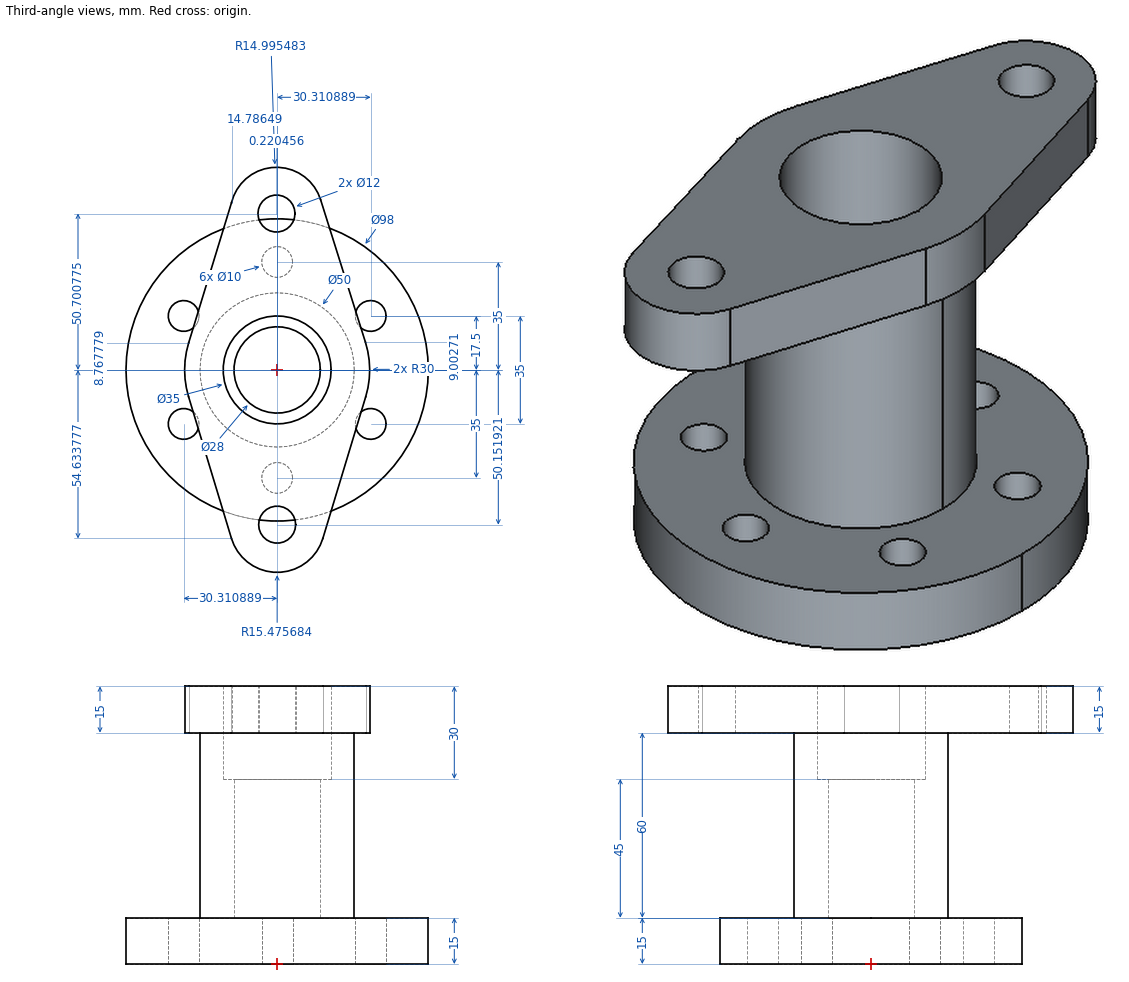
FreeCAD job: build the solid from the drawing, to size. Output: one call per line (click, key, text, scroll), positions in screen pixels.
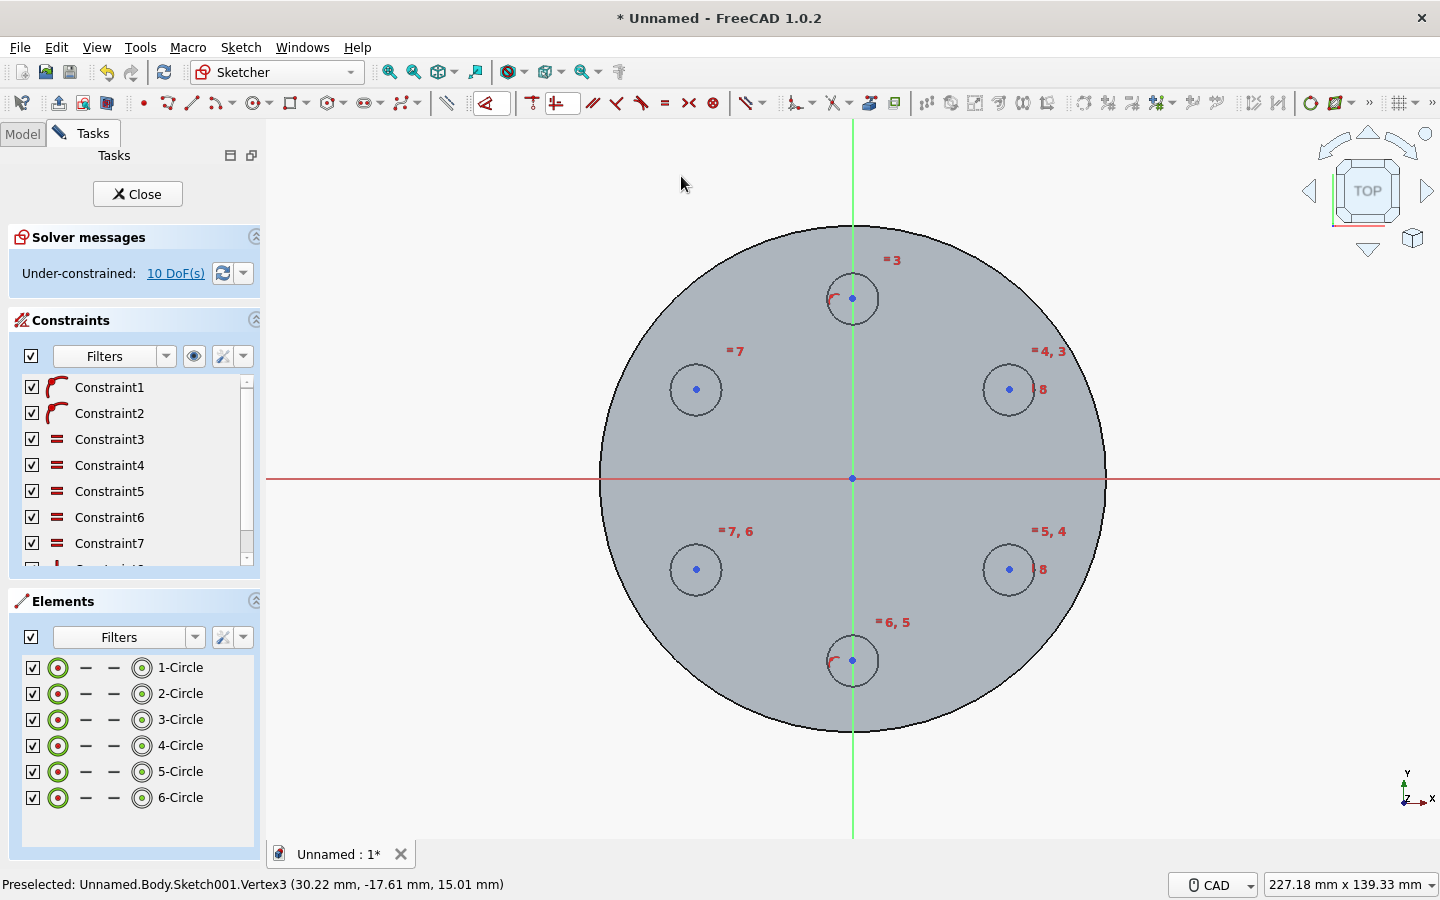
click(1009, 570)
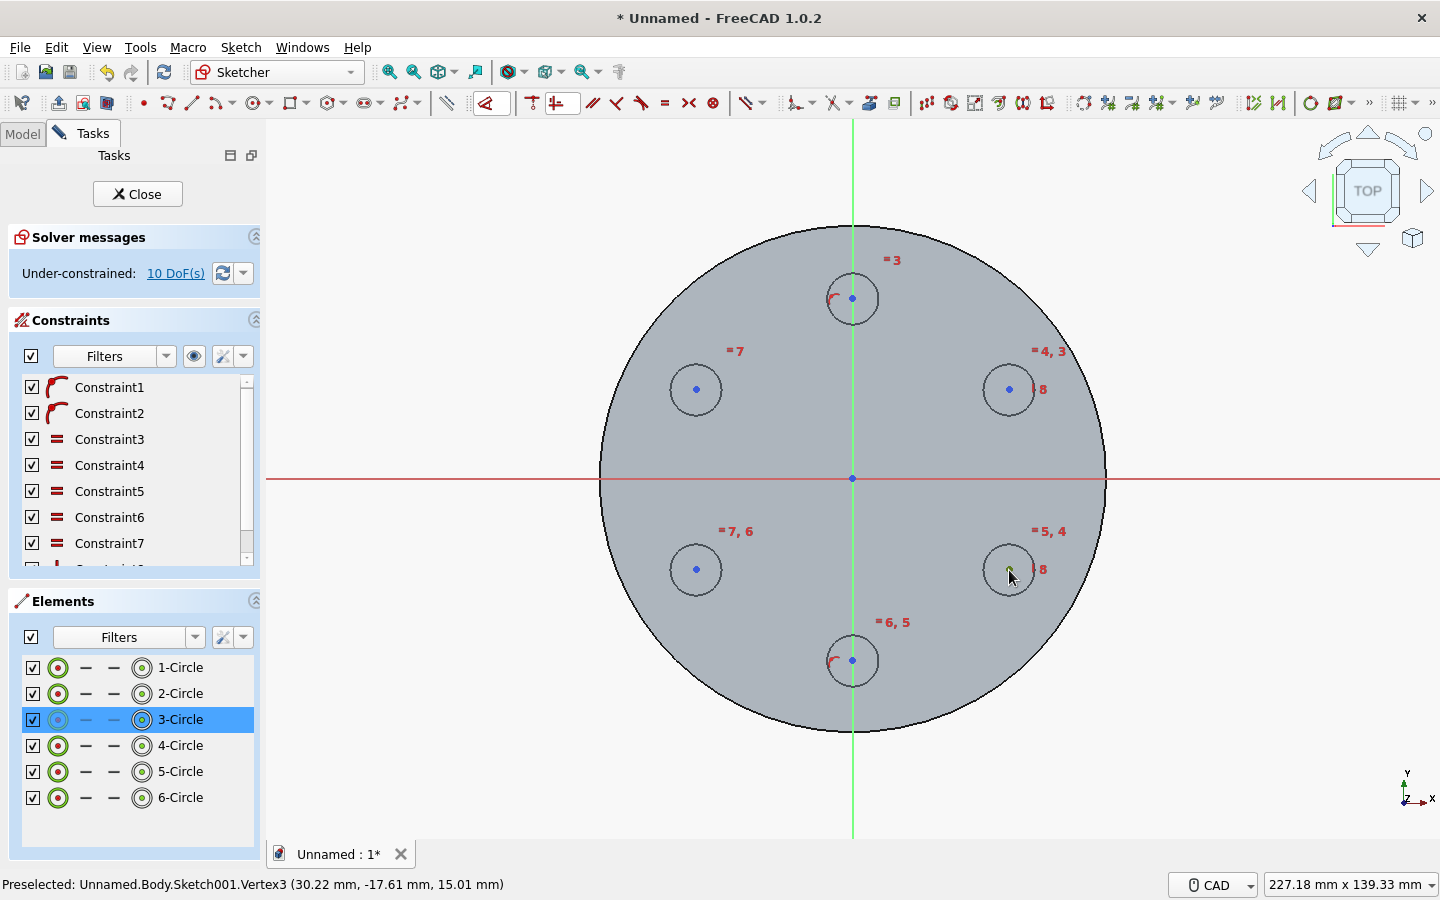
click(696, 570)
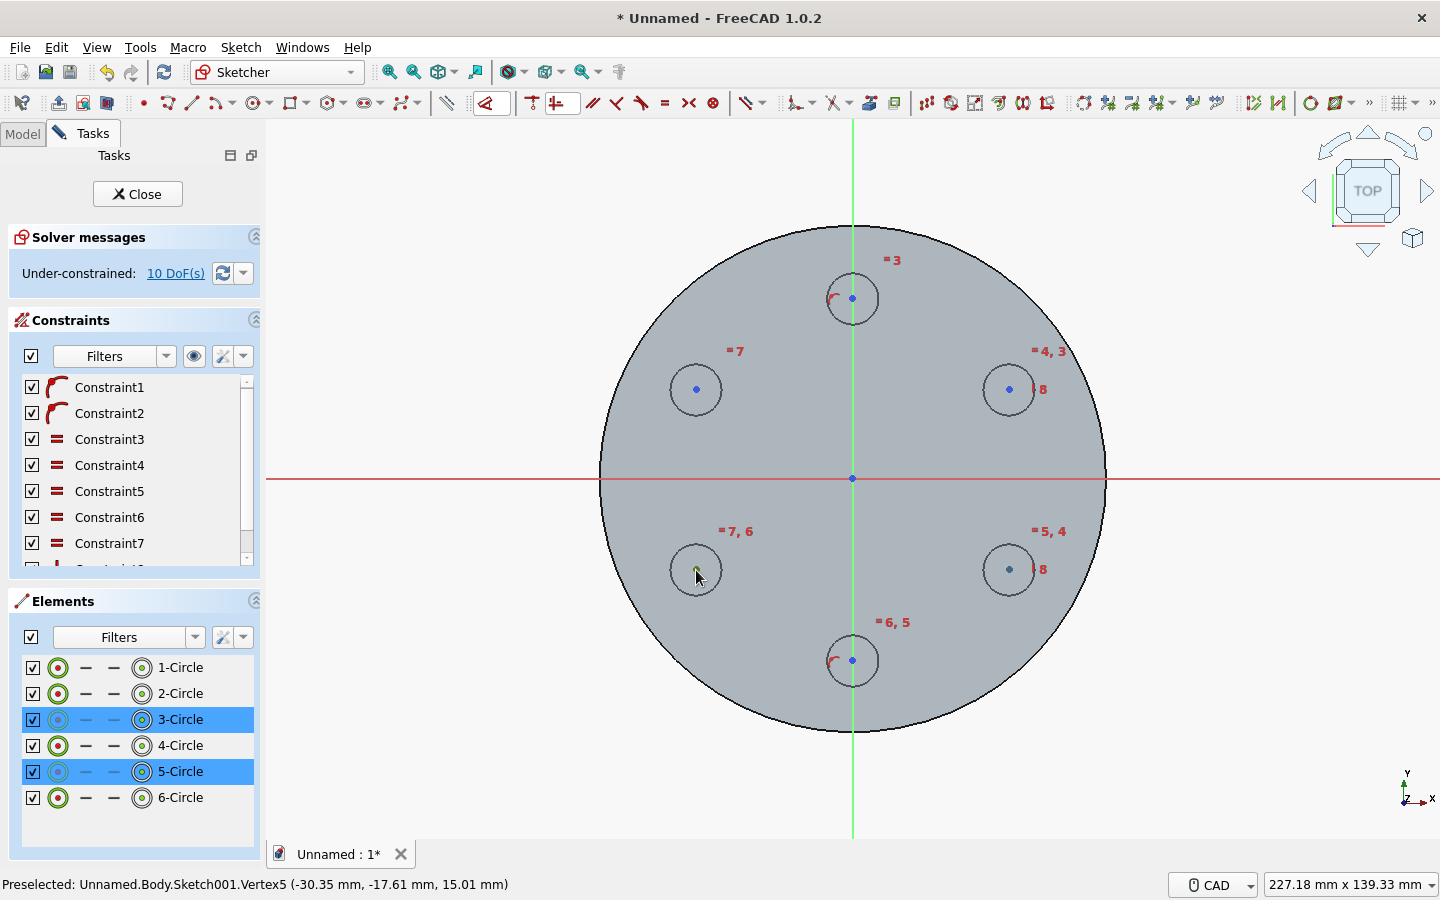
key(h)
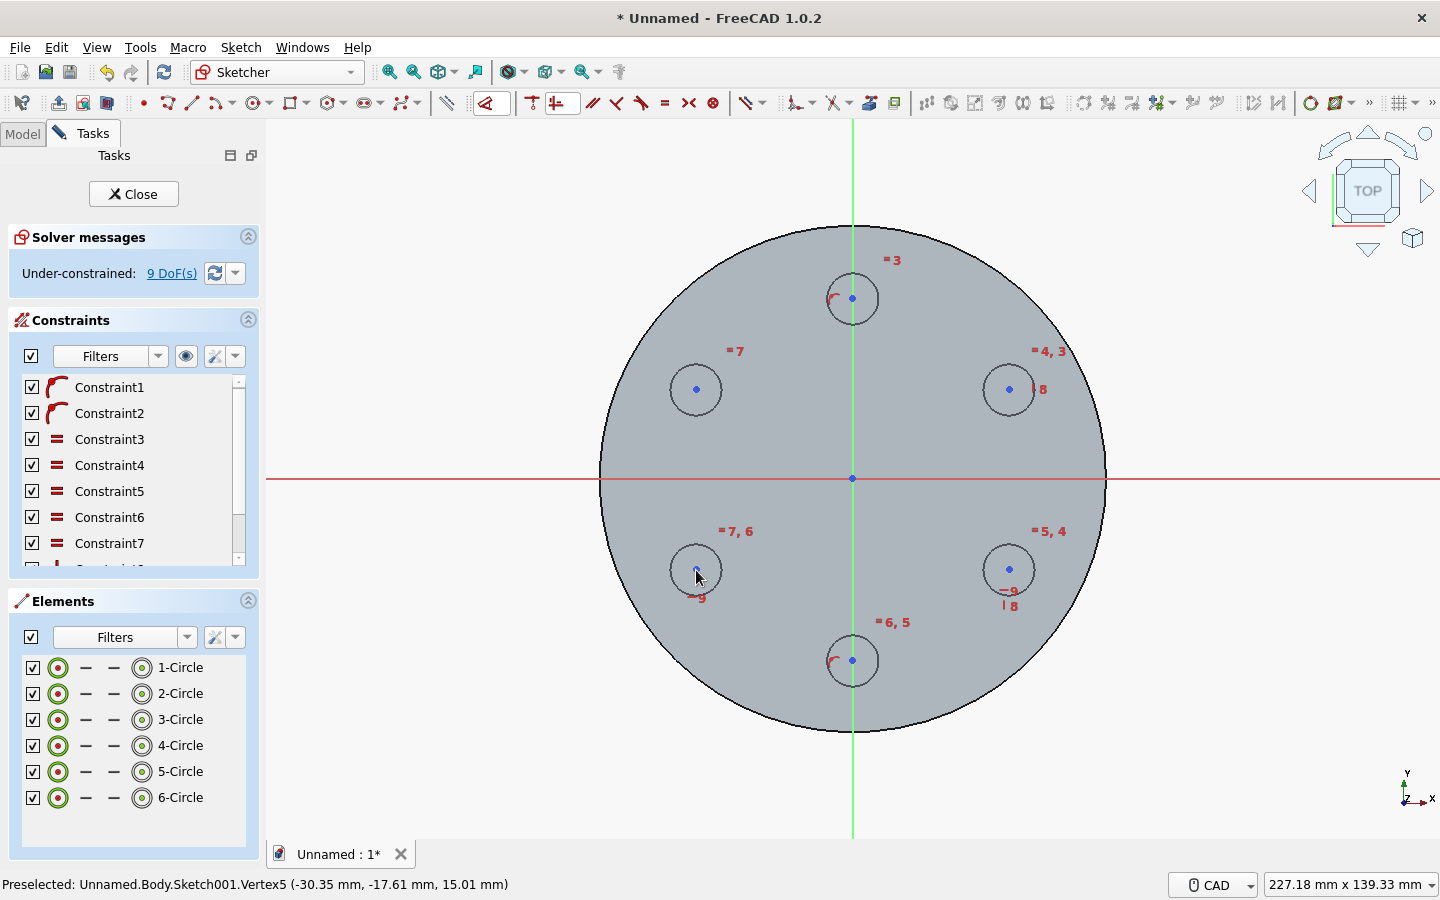
click(696, 570)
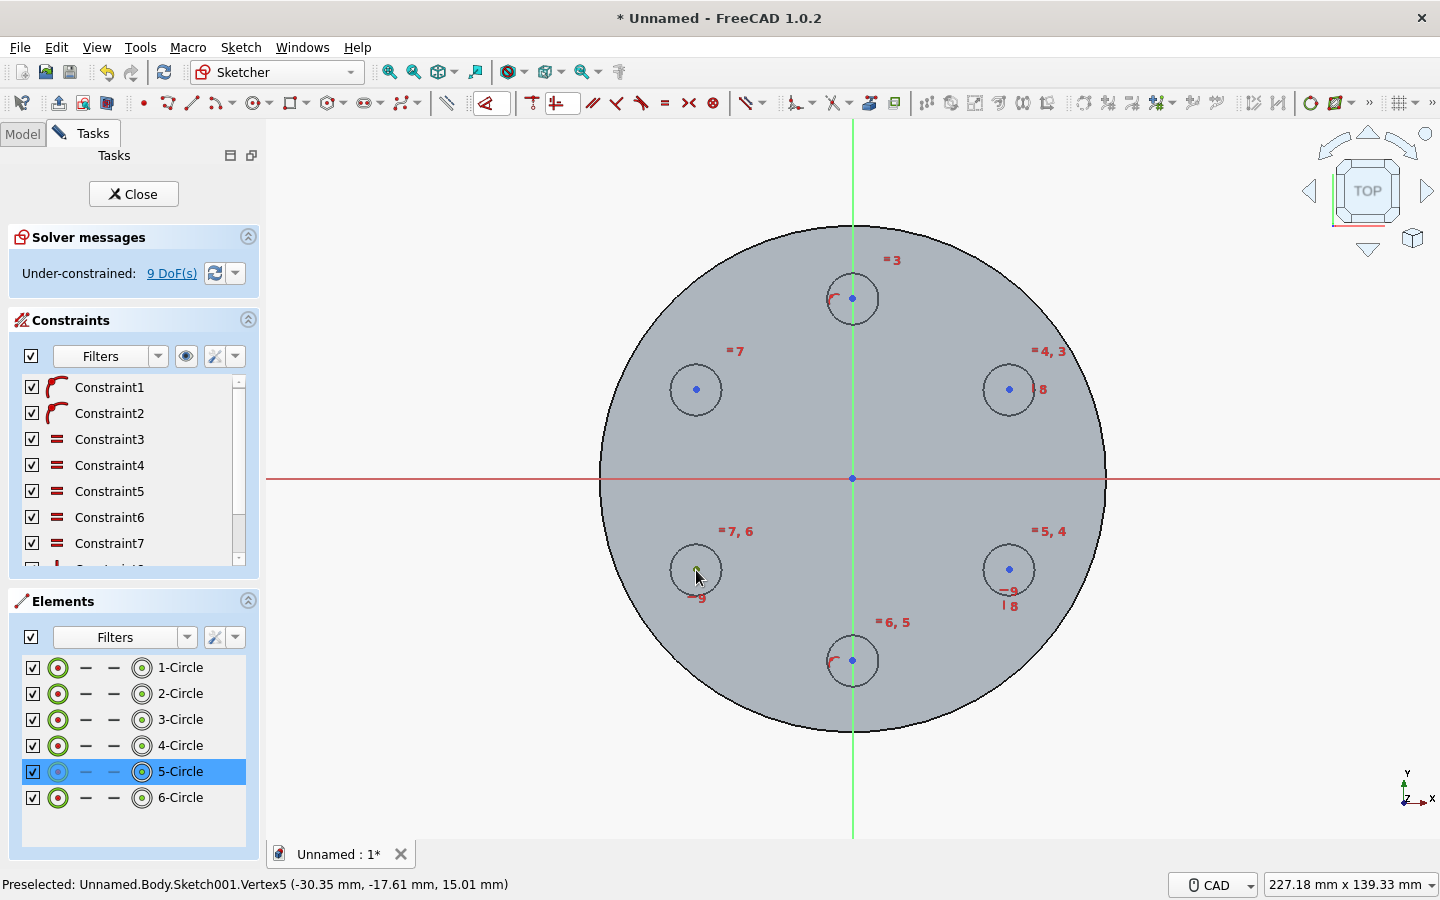
click(696, 390)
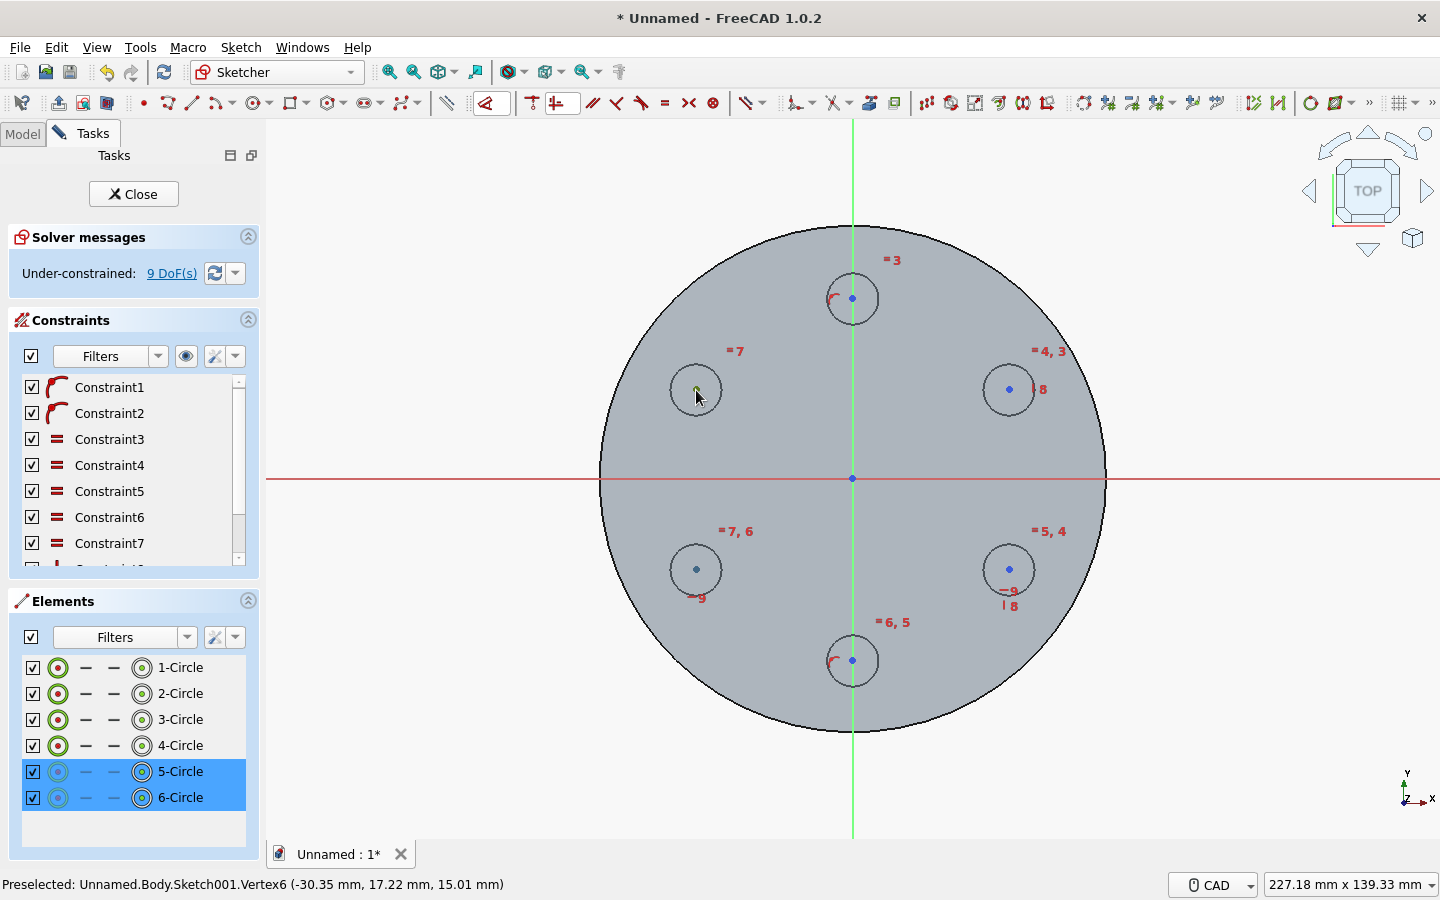
click(574, 104)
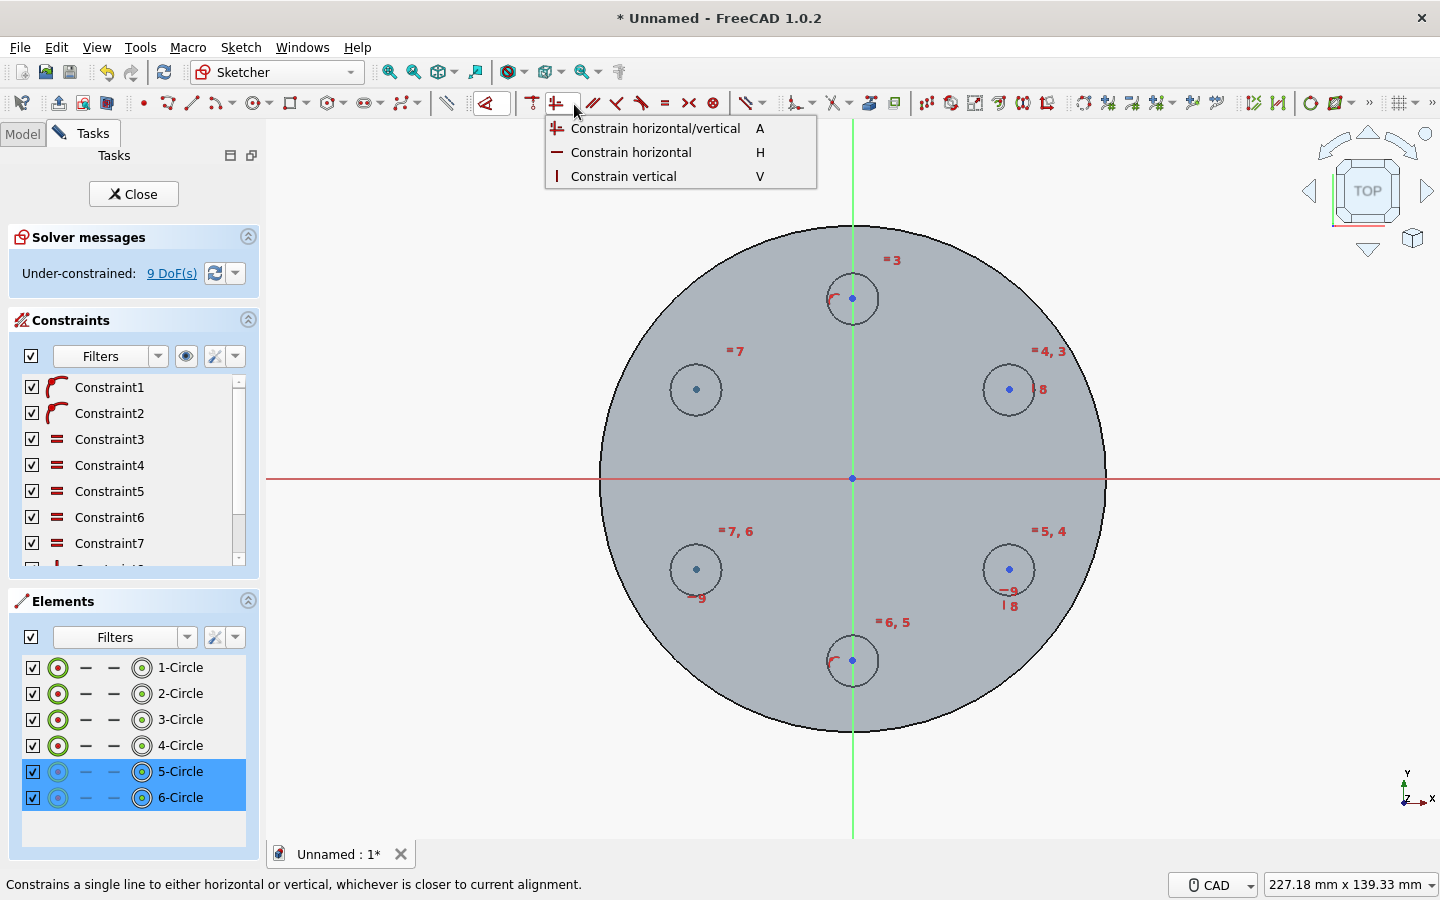
click(681, 176)